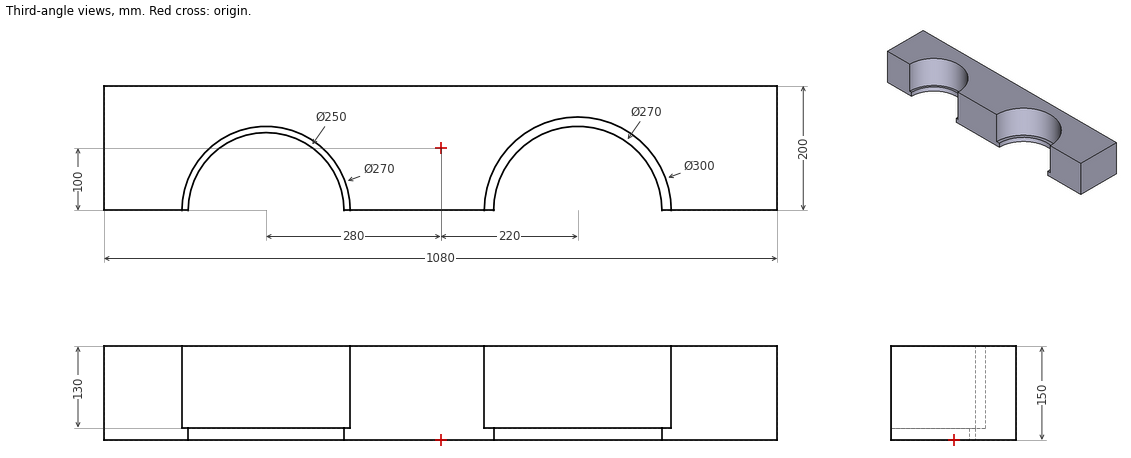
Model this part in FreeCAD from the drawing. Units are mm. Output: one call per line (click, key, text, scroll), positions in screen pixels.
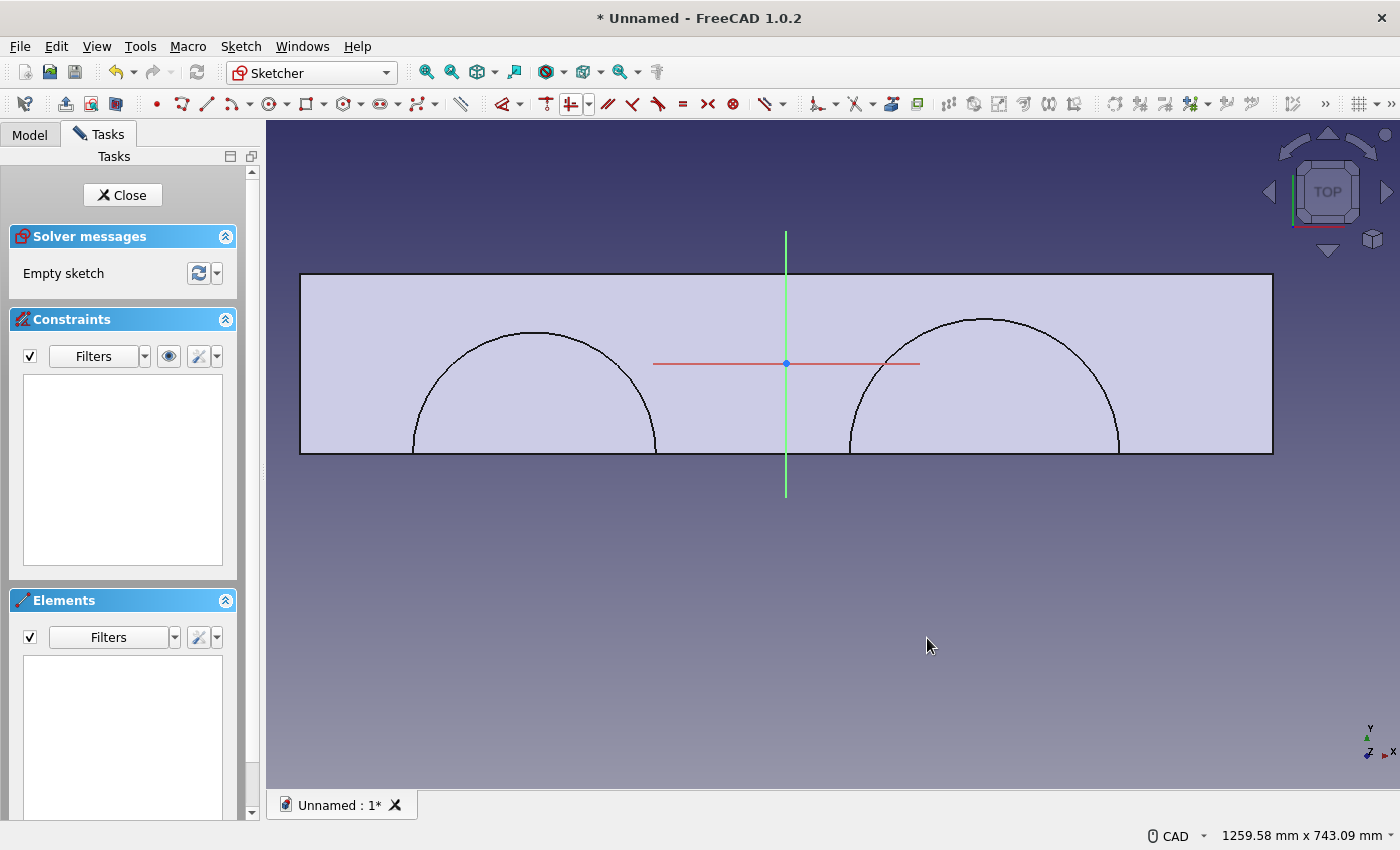
key(g)
key(c)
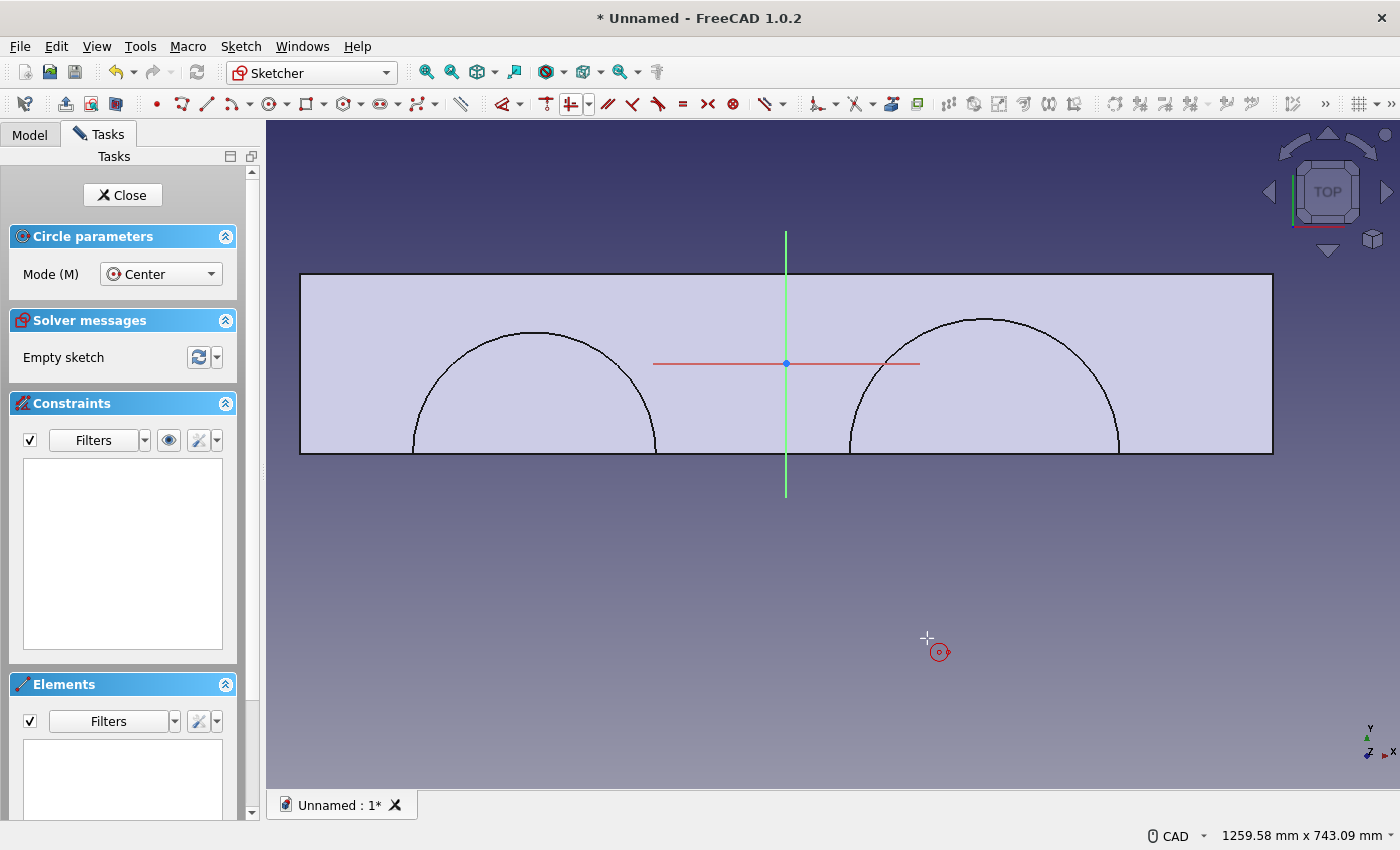
click(534, 454)
click(614, 533)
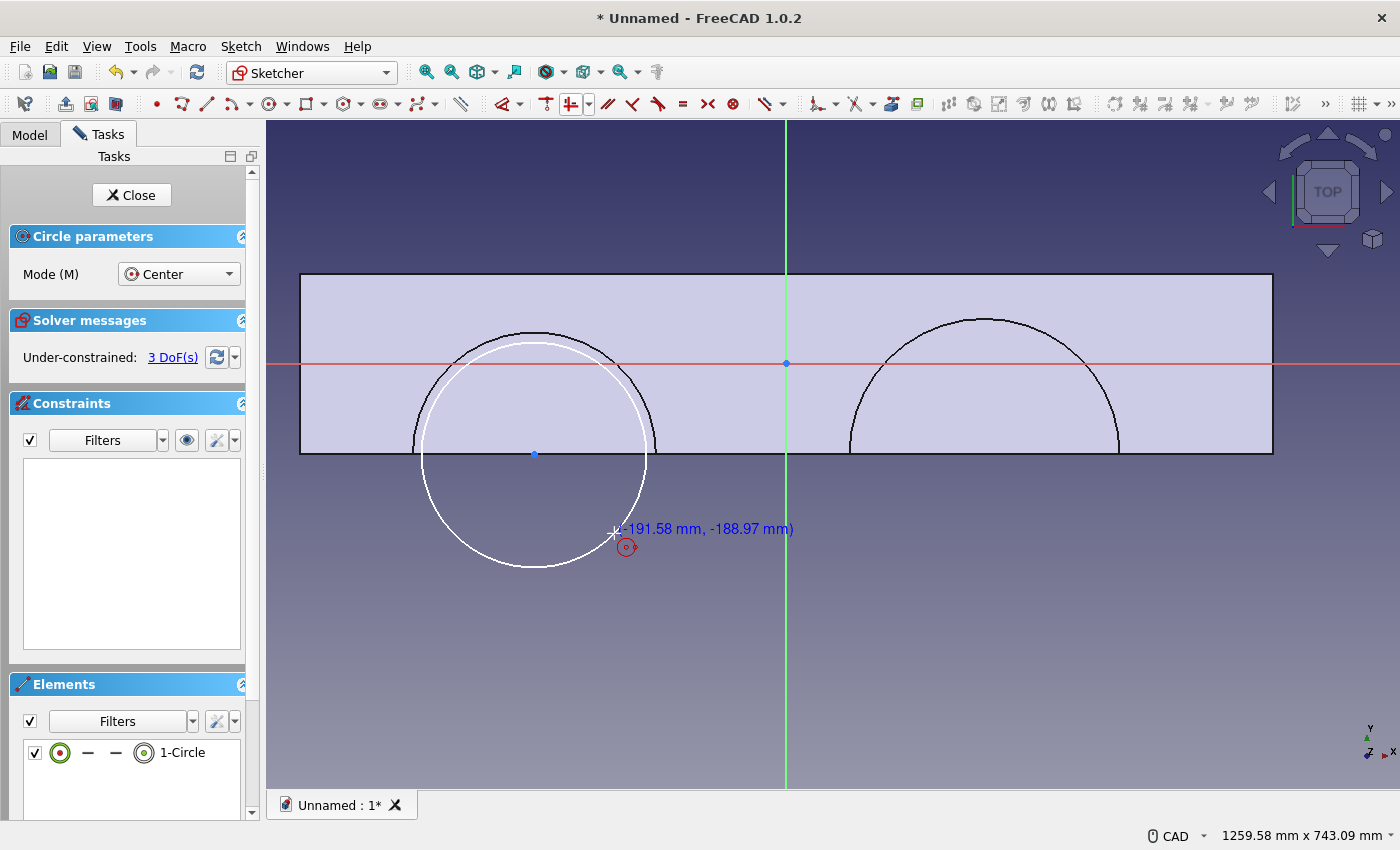
click(985, 454)
click(1070, 540)
key(Escape)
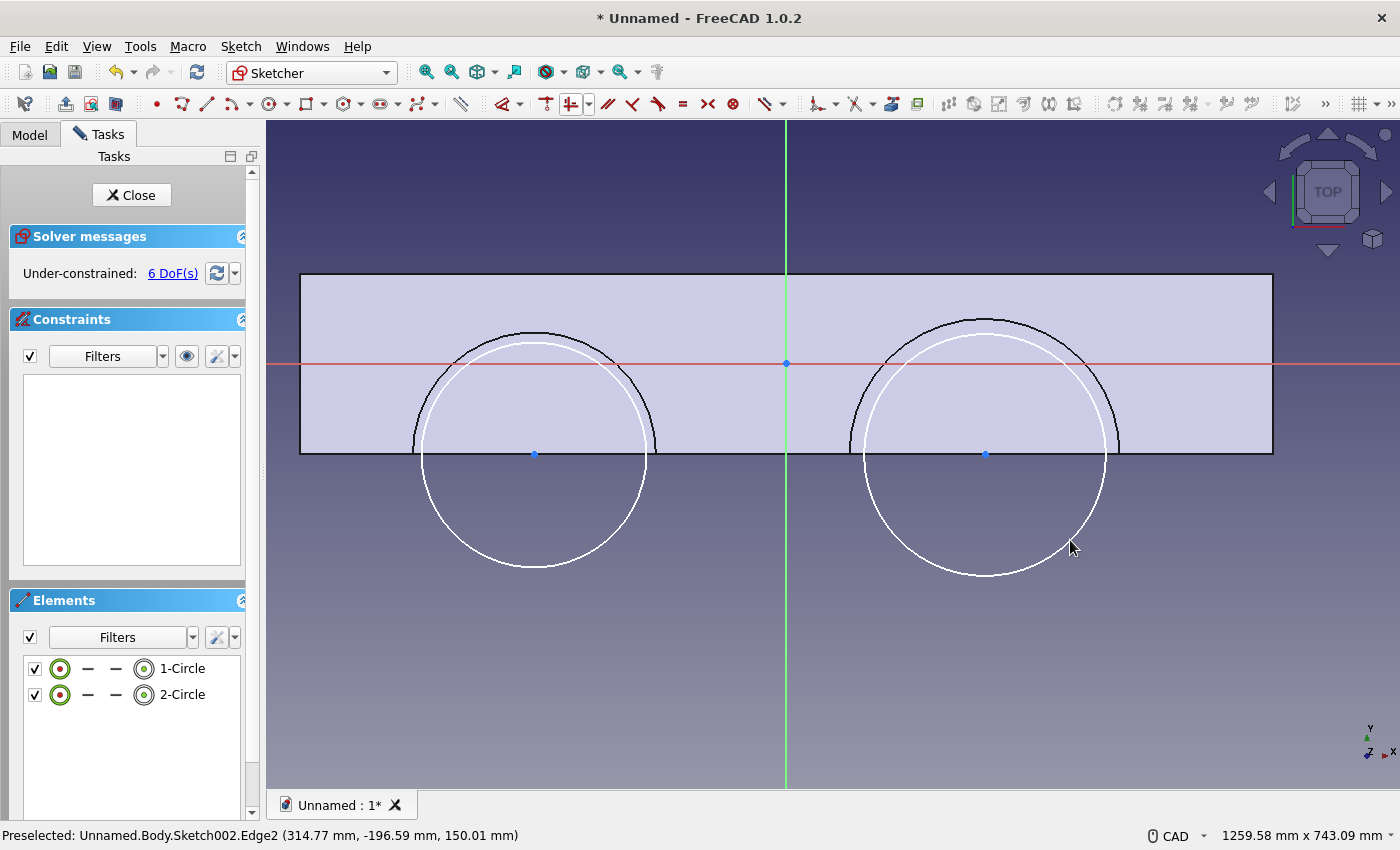
click(534, 455)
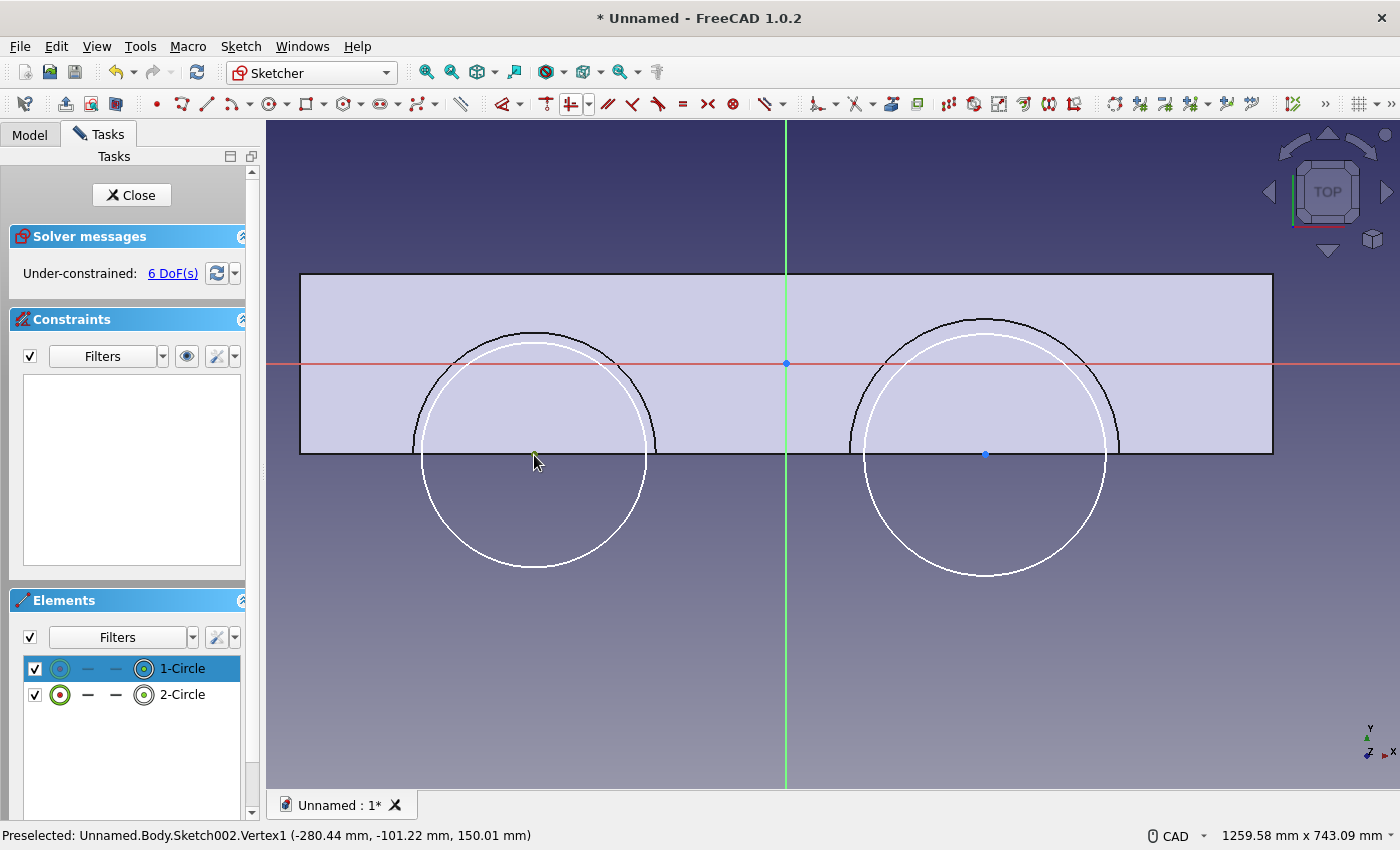
click(985, 455)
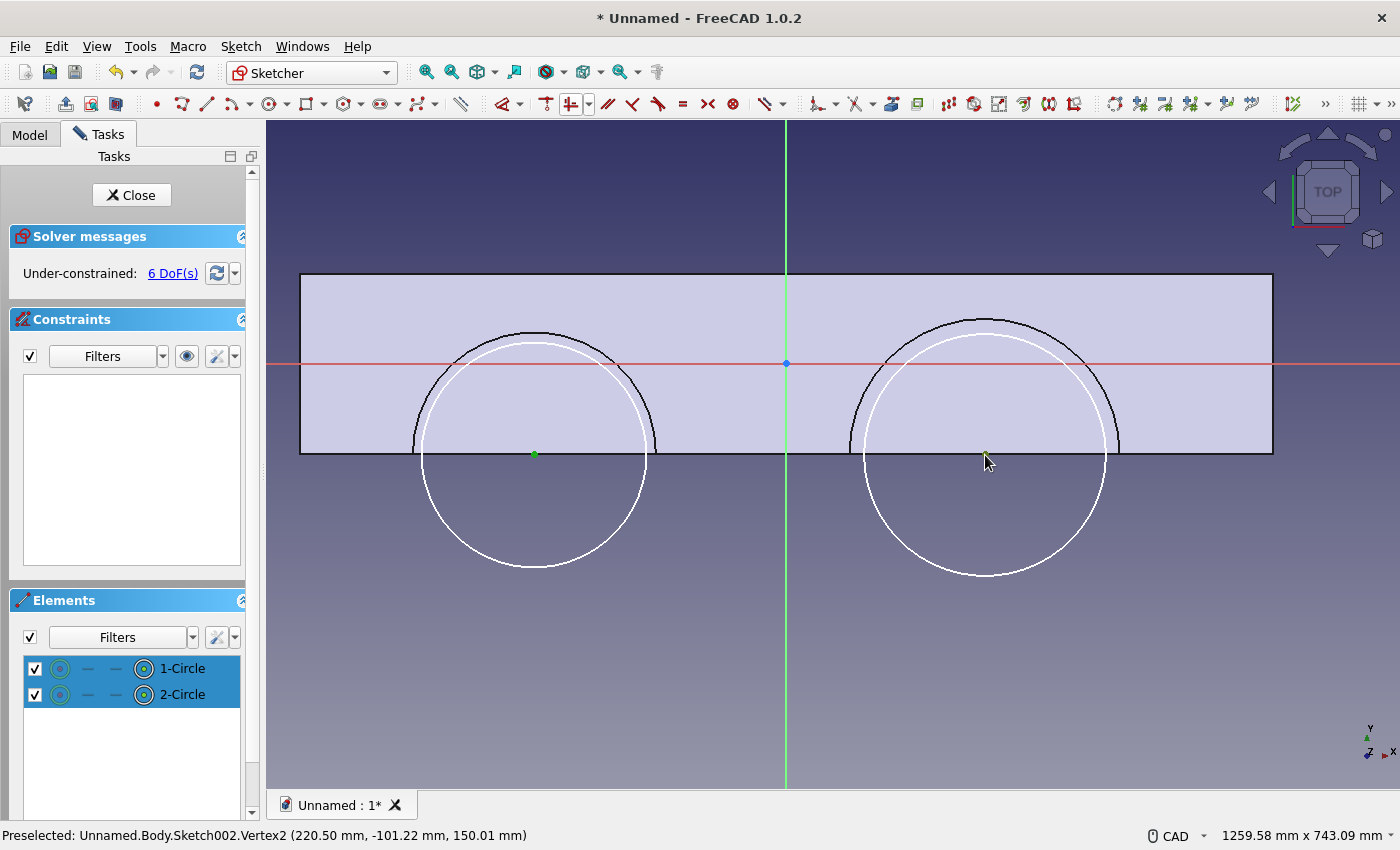
key(h)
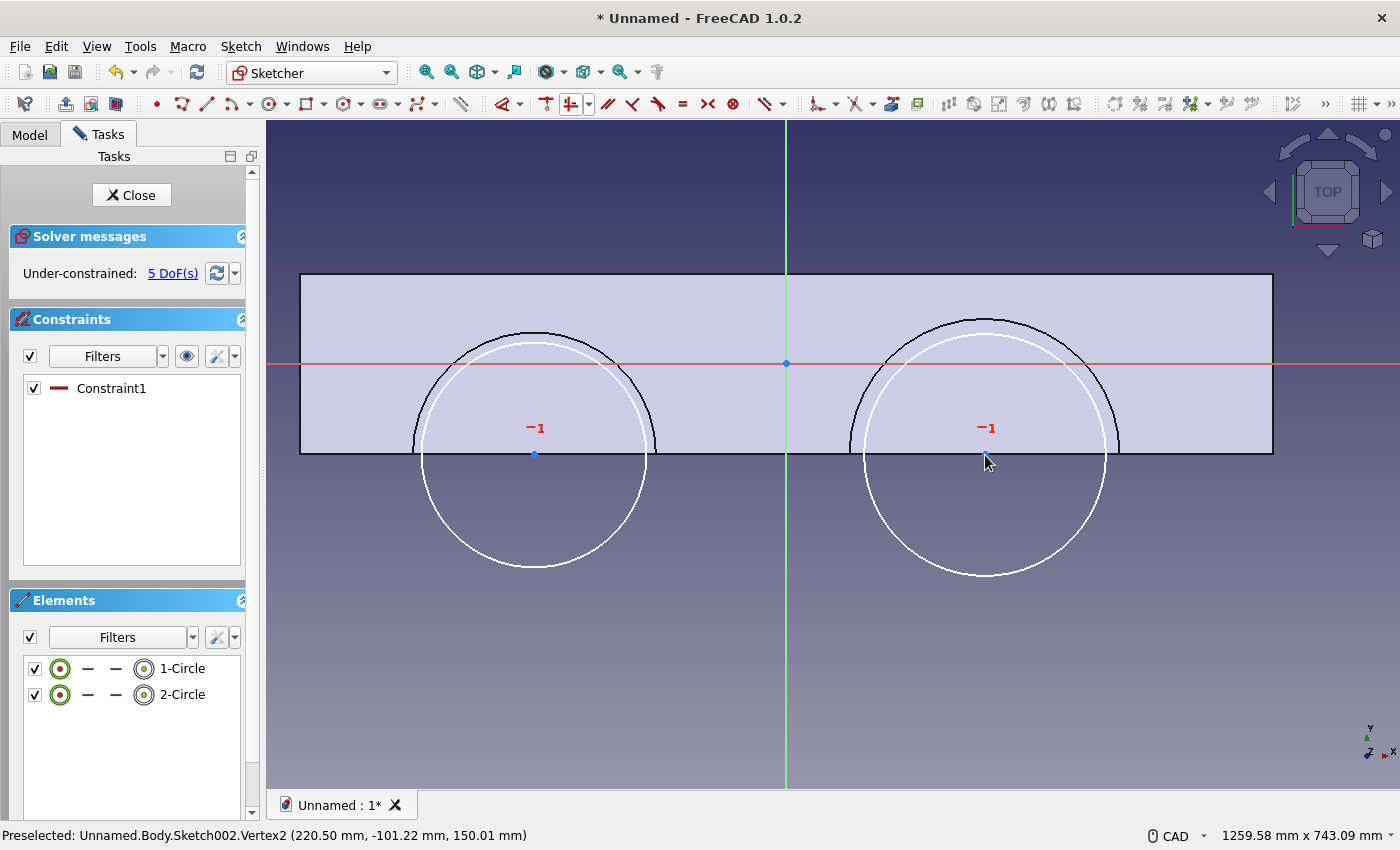
key(d)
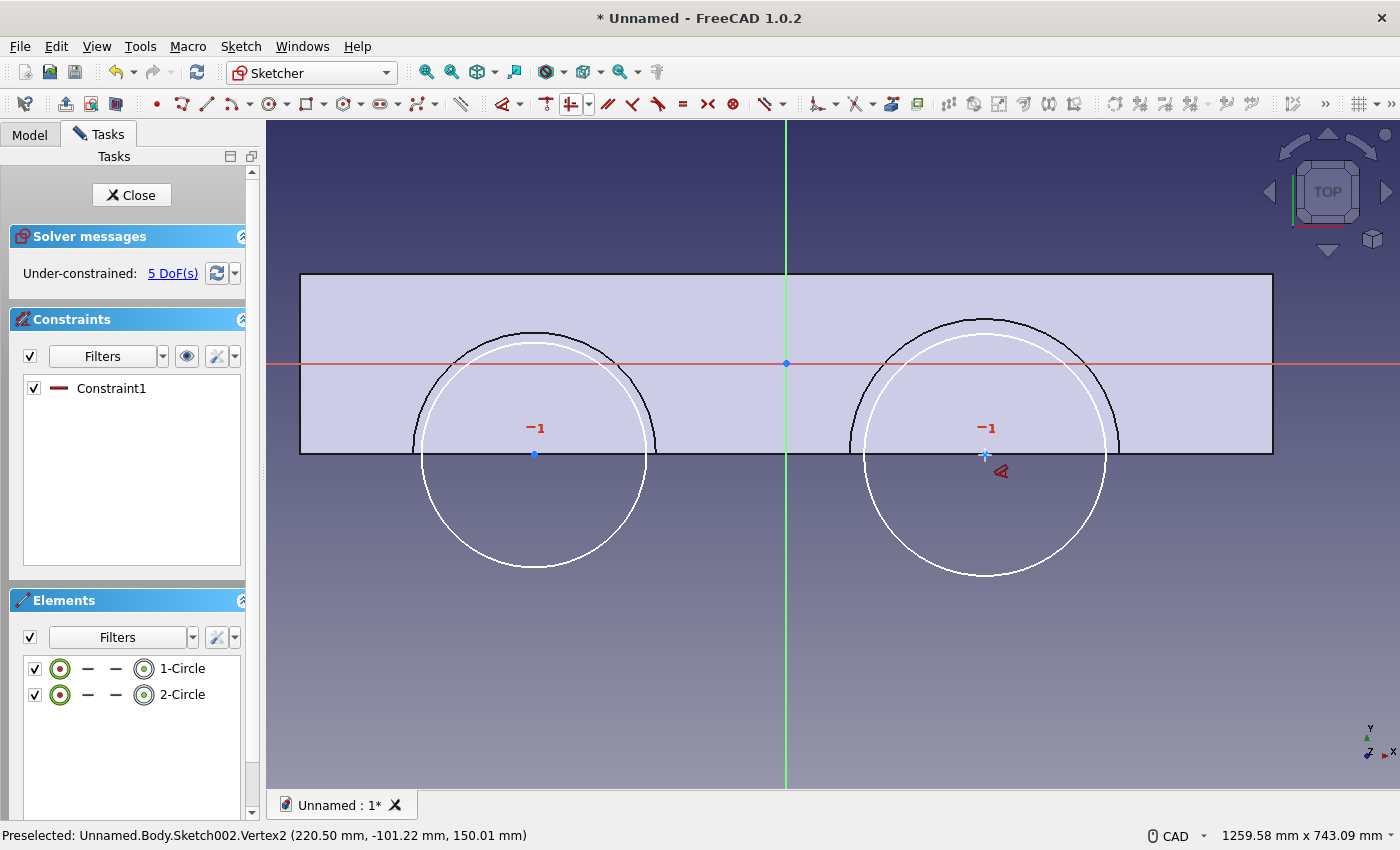
click(613, 375)
click(672, 413)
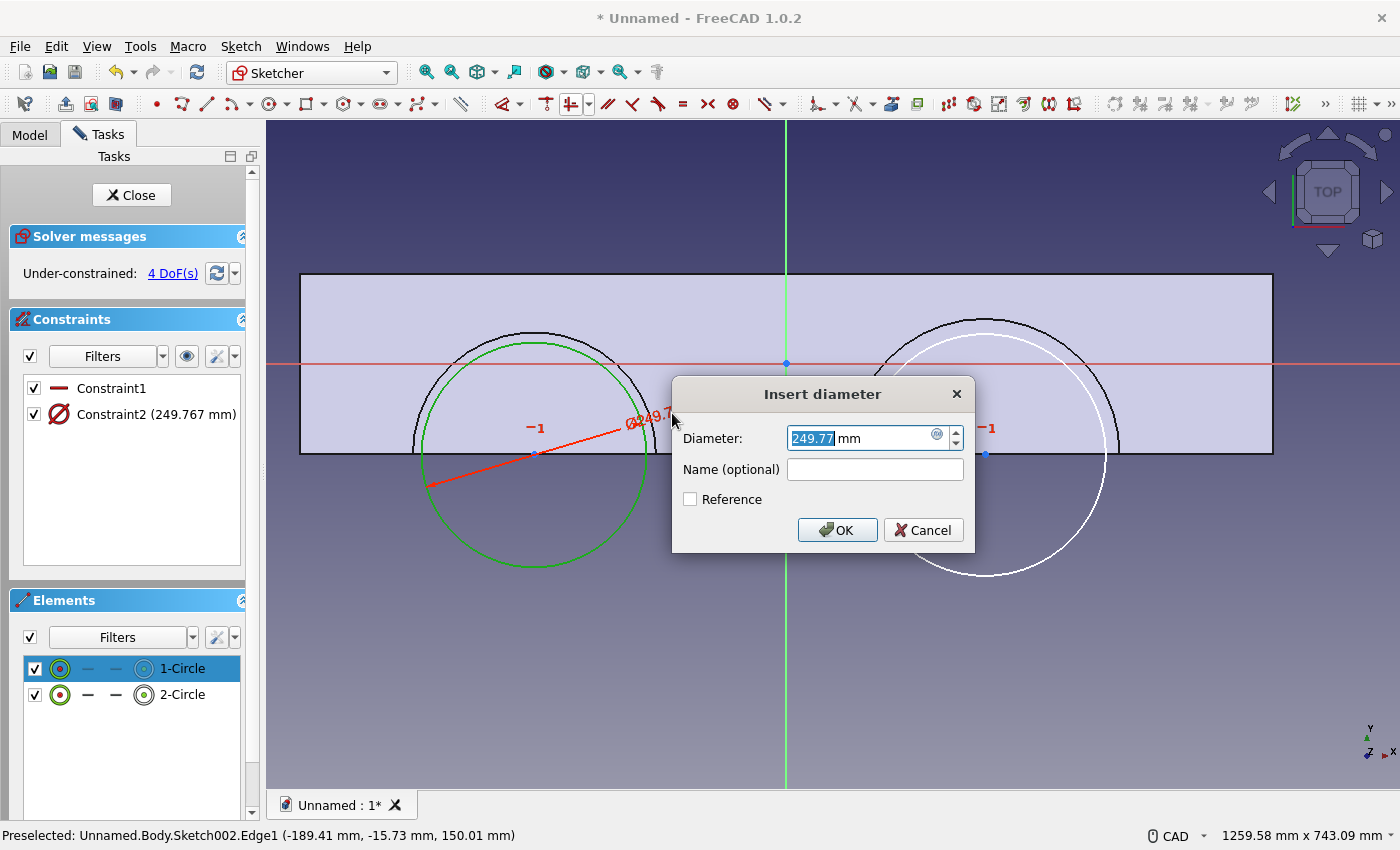
text(250)
key(Return)